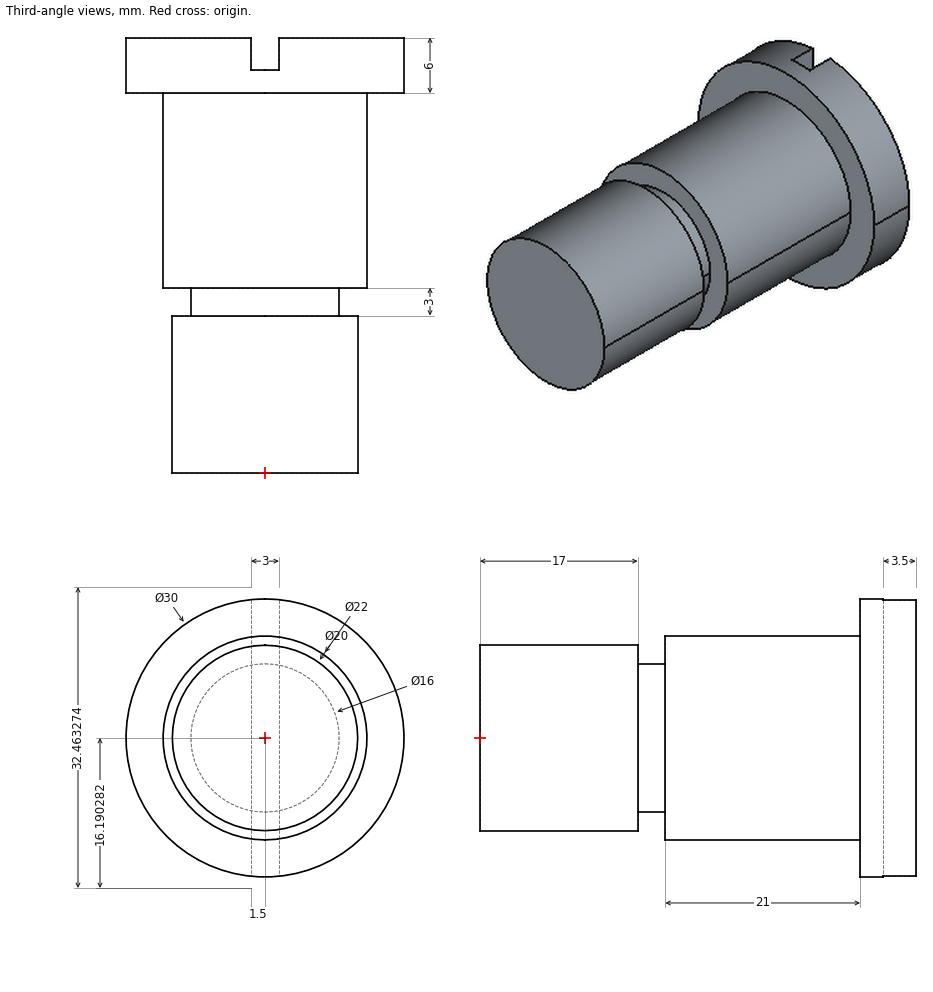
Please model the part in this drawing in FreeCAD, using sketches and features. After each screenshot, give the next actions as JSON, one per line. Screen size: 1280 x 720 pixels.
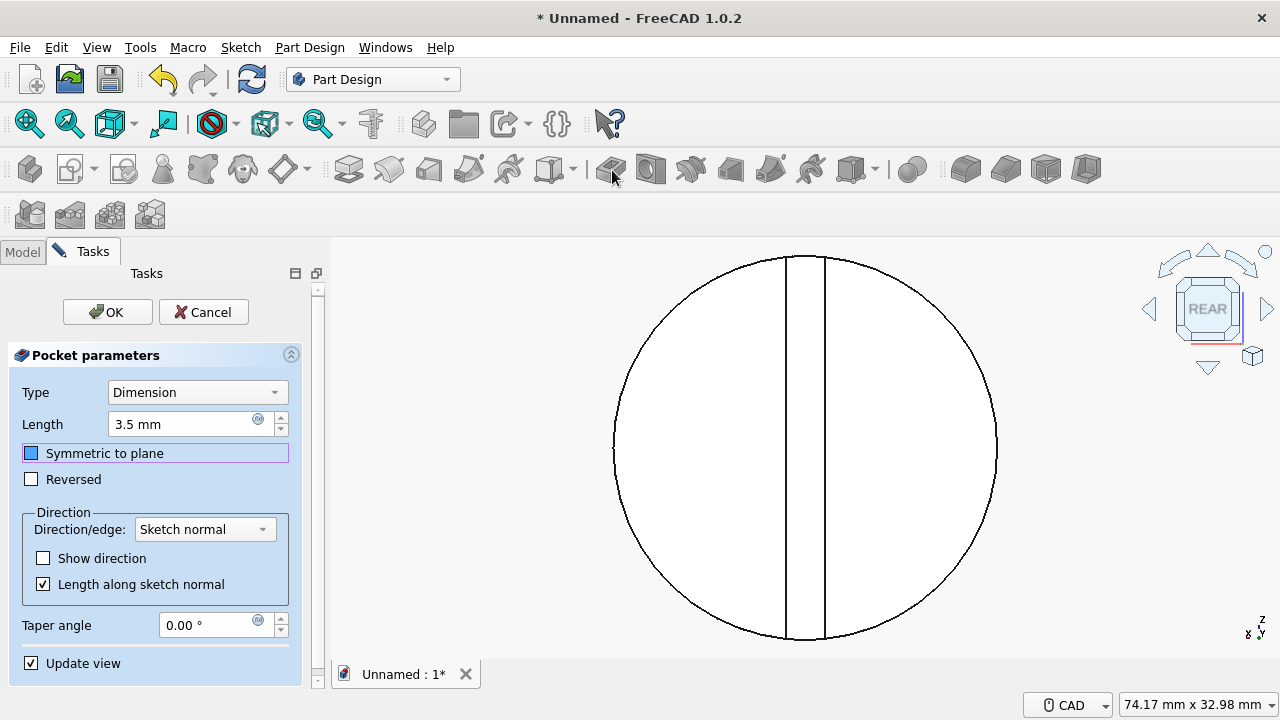
{"action": "left_click", "coordinate": [108, 312]}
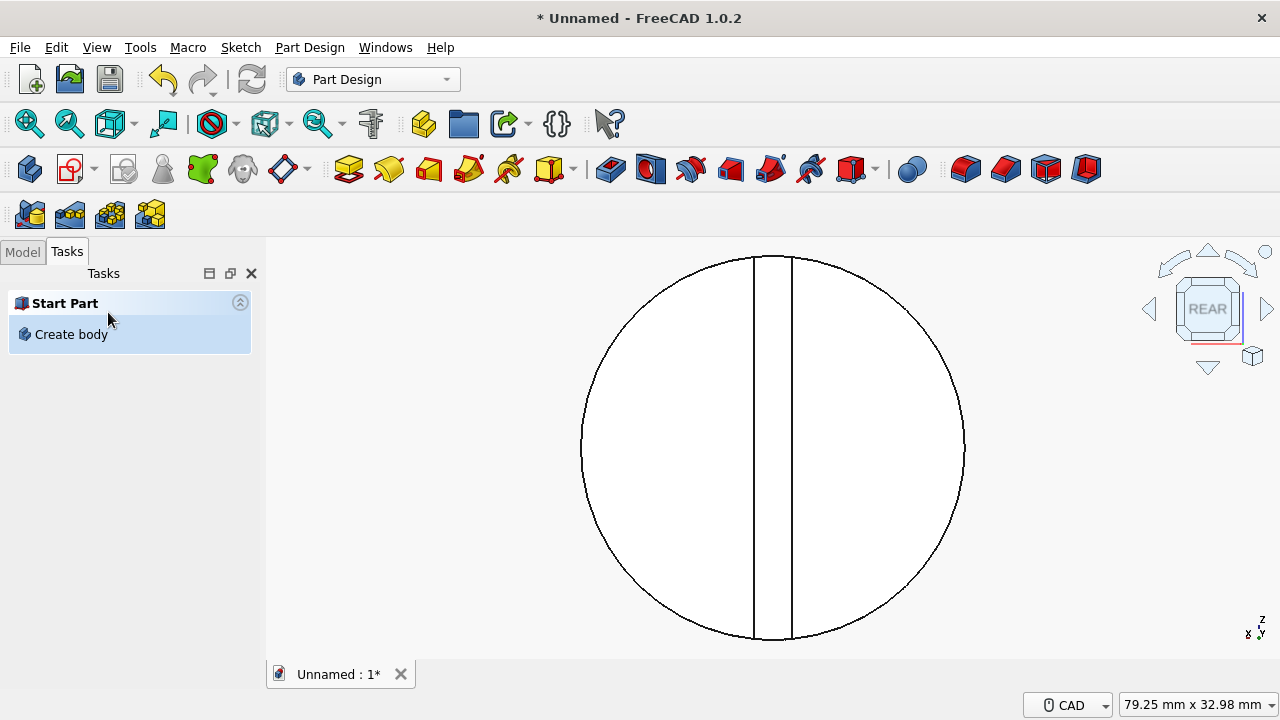
{"action": "key", "text": "0"}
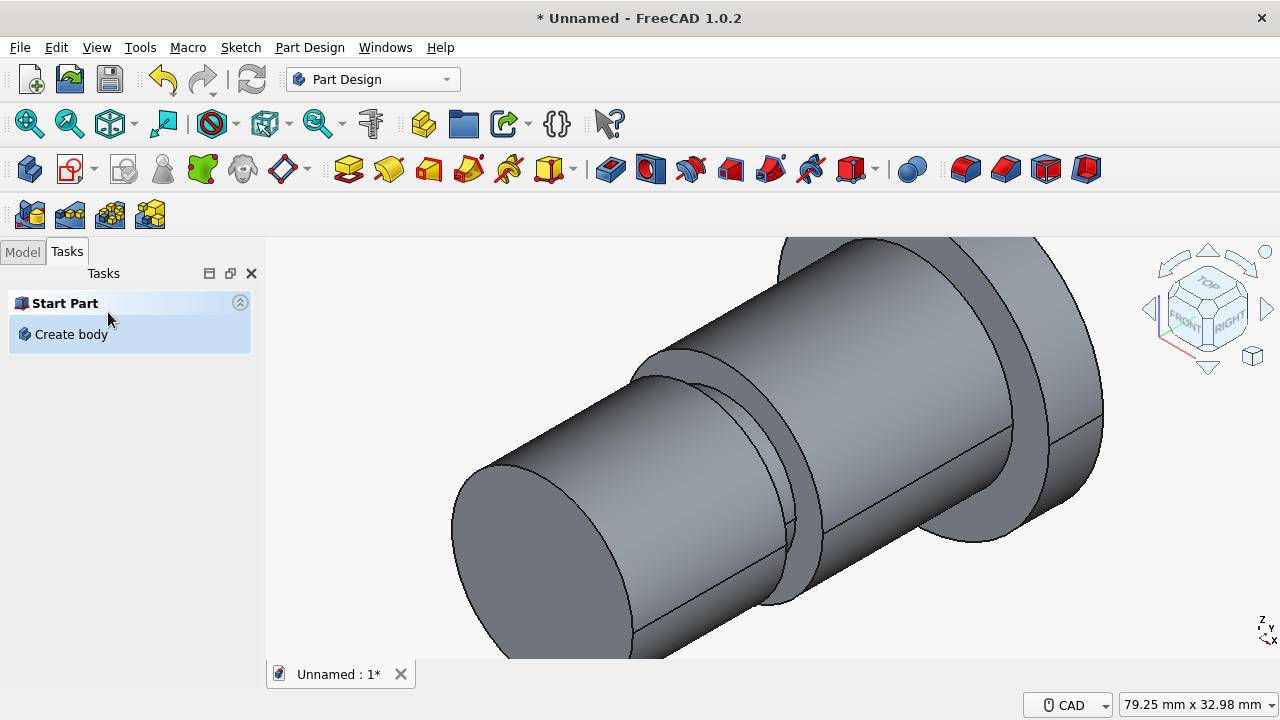
{"action": "left_click", "coordinate": [30, 124]}